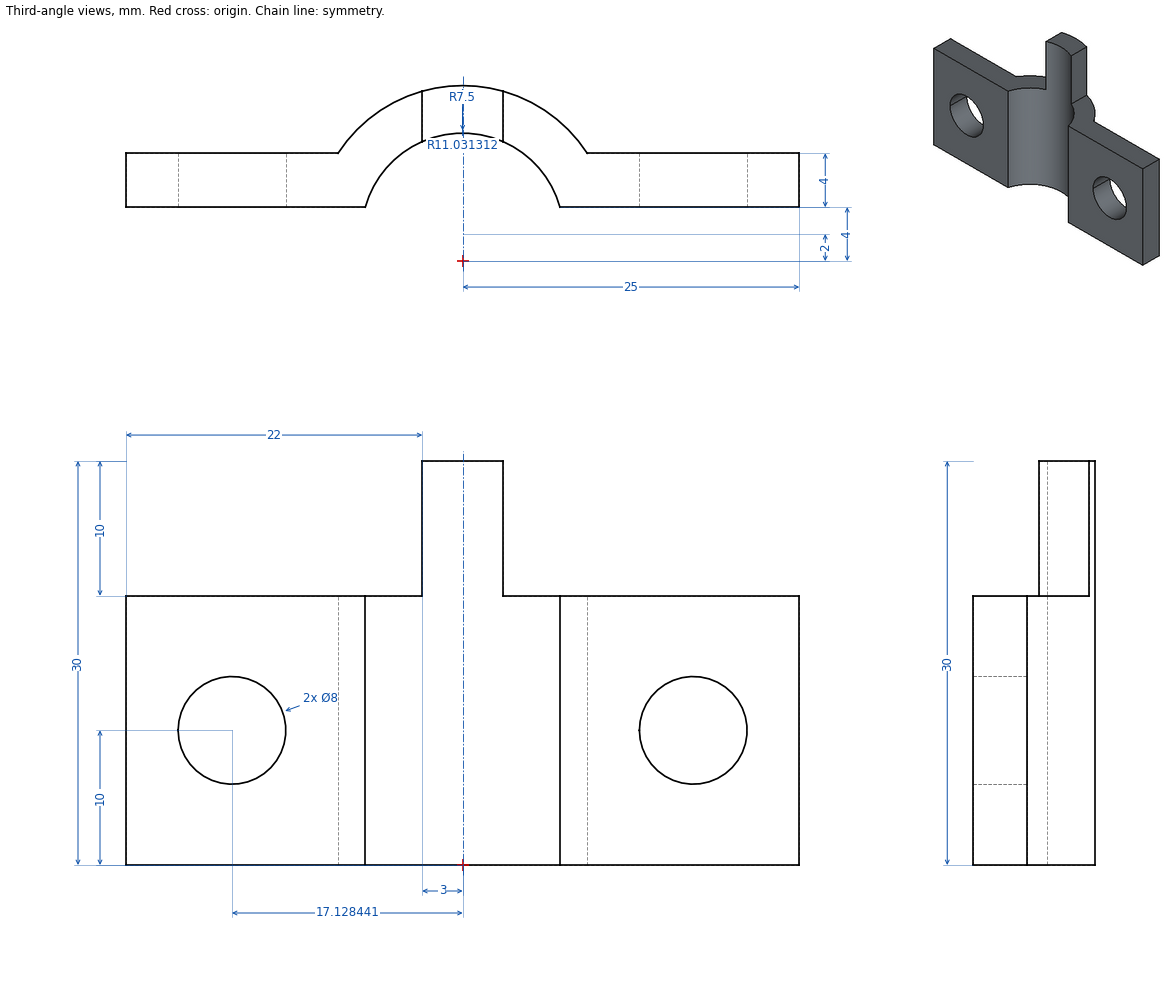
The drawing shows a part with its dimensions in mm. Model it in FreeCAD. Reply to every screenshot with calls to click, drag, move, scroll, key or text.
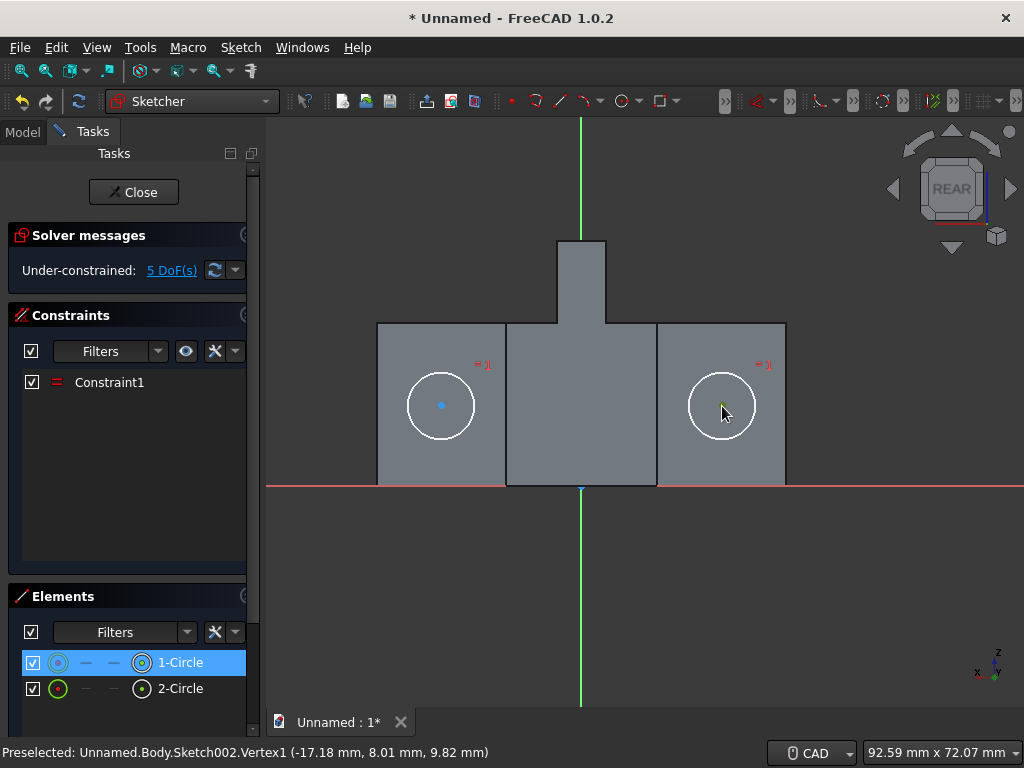
click(441, 406)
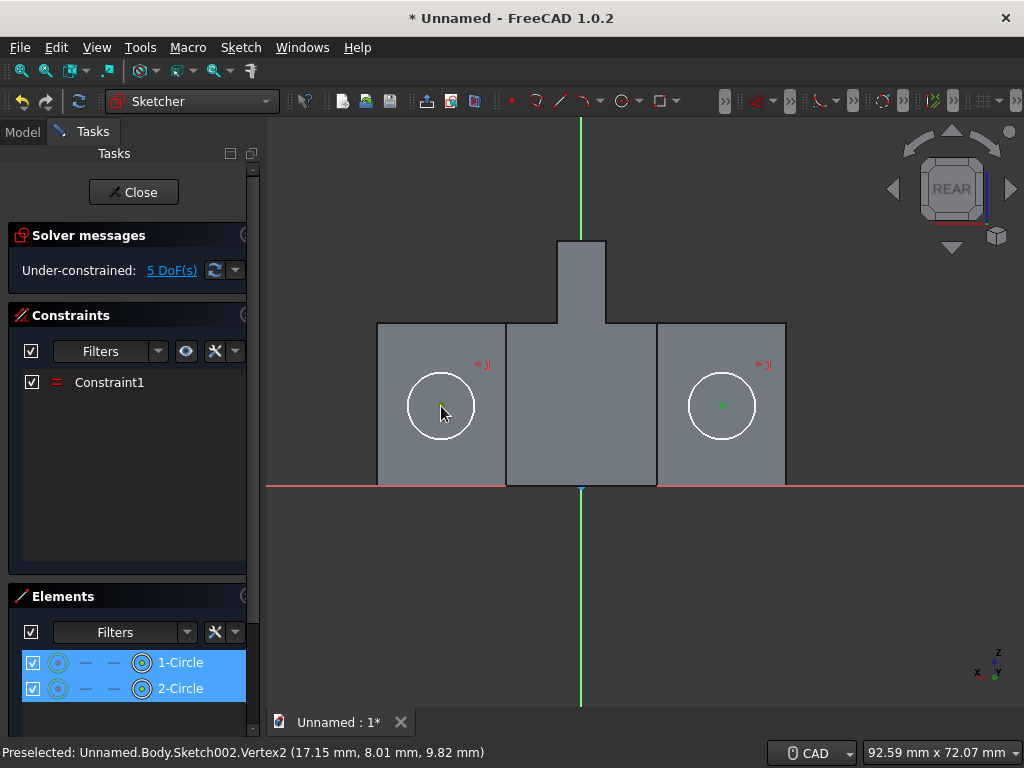
click(581, 641)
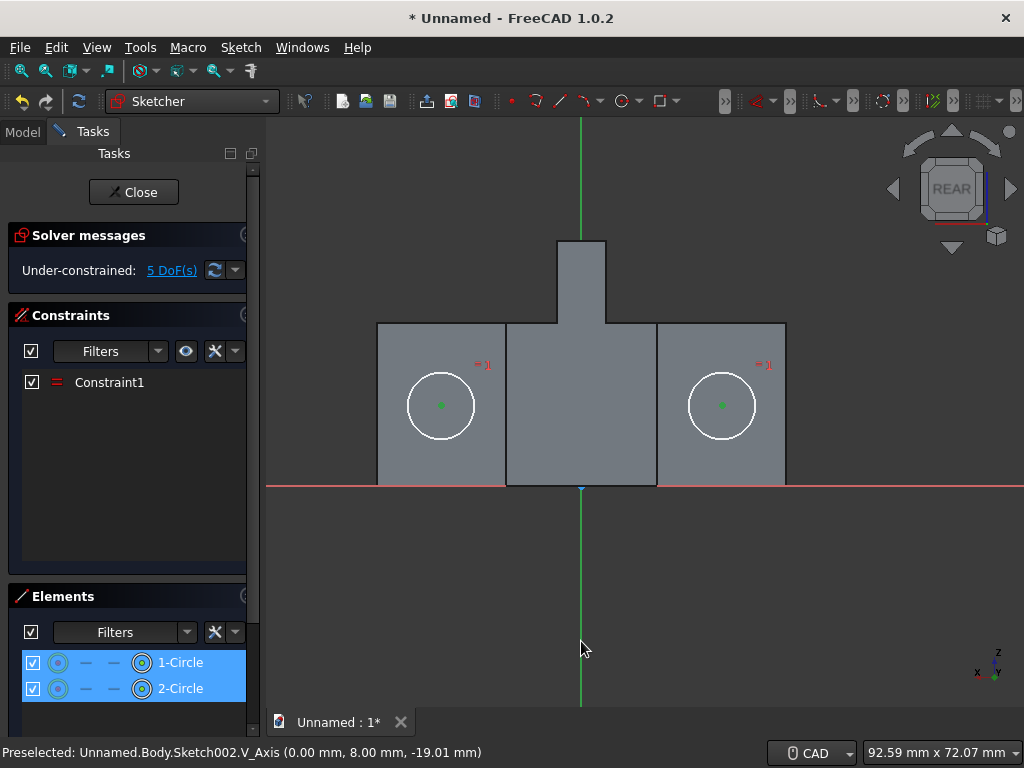
key(s)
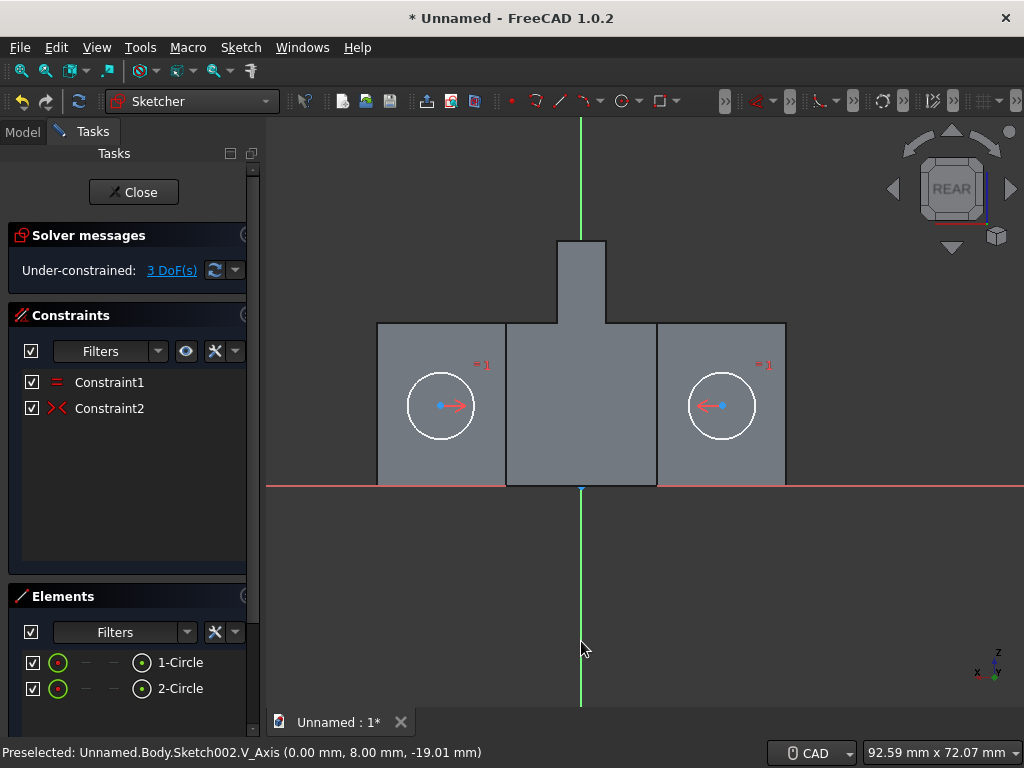
click(756, 102)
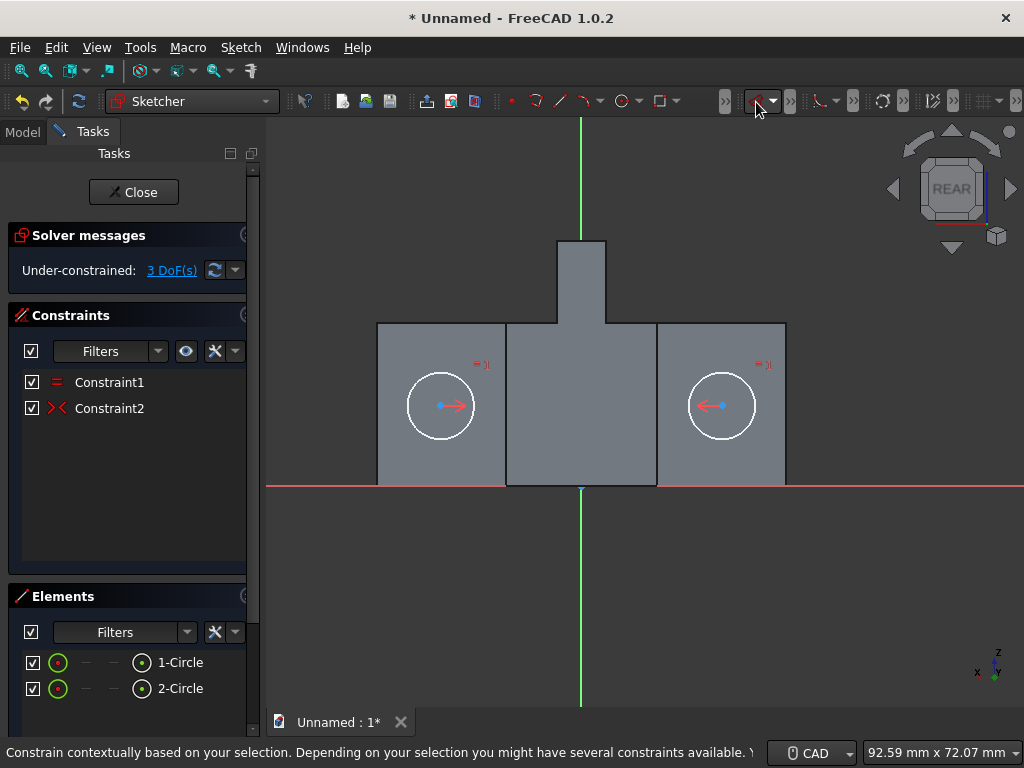
click(745, 382)
click(767, 359)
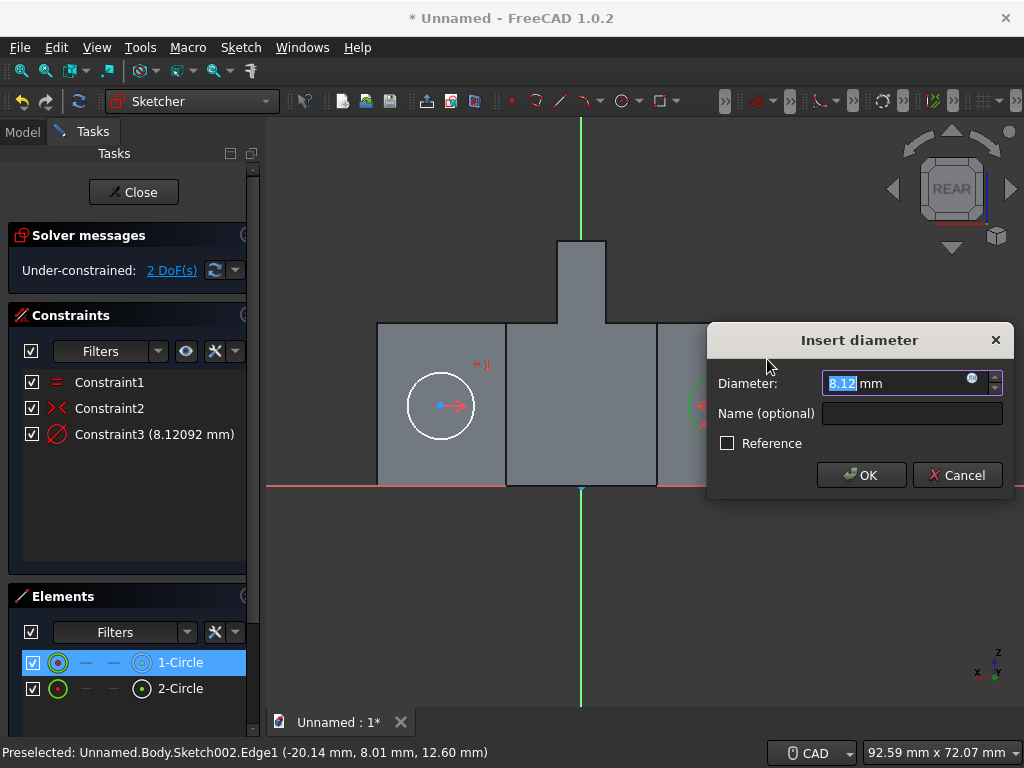
text(8)
key(Return)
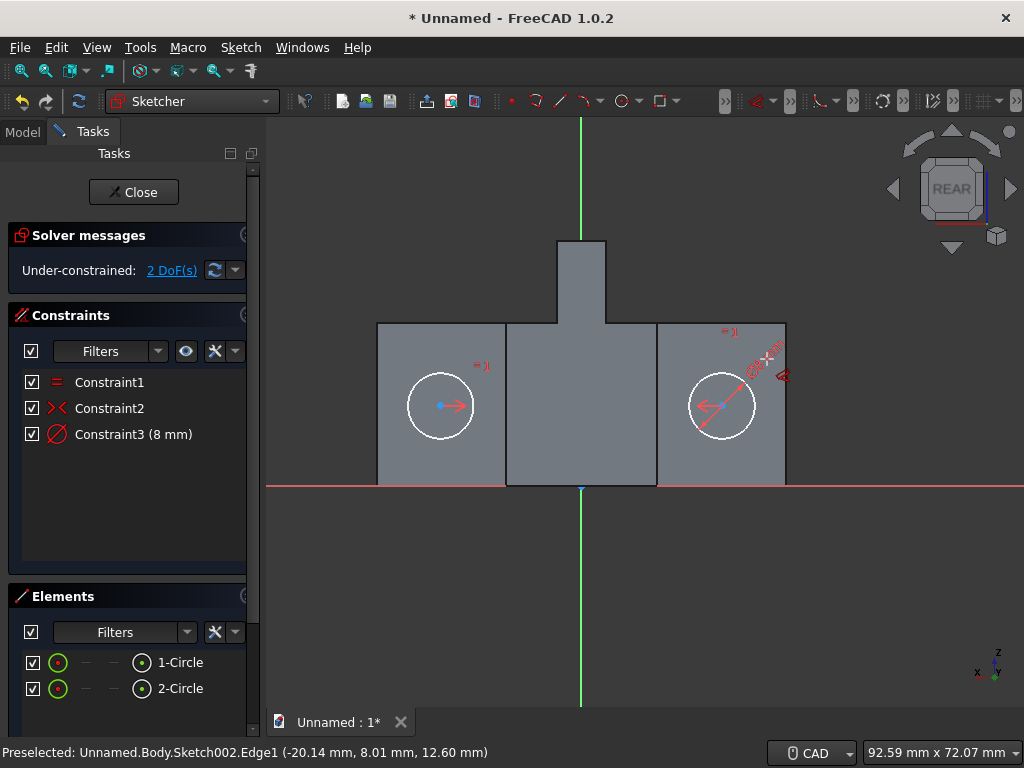
click(722, 406)
click(756, 446)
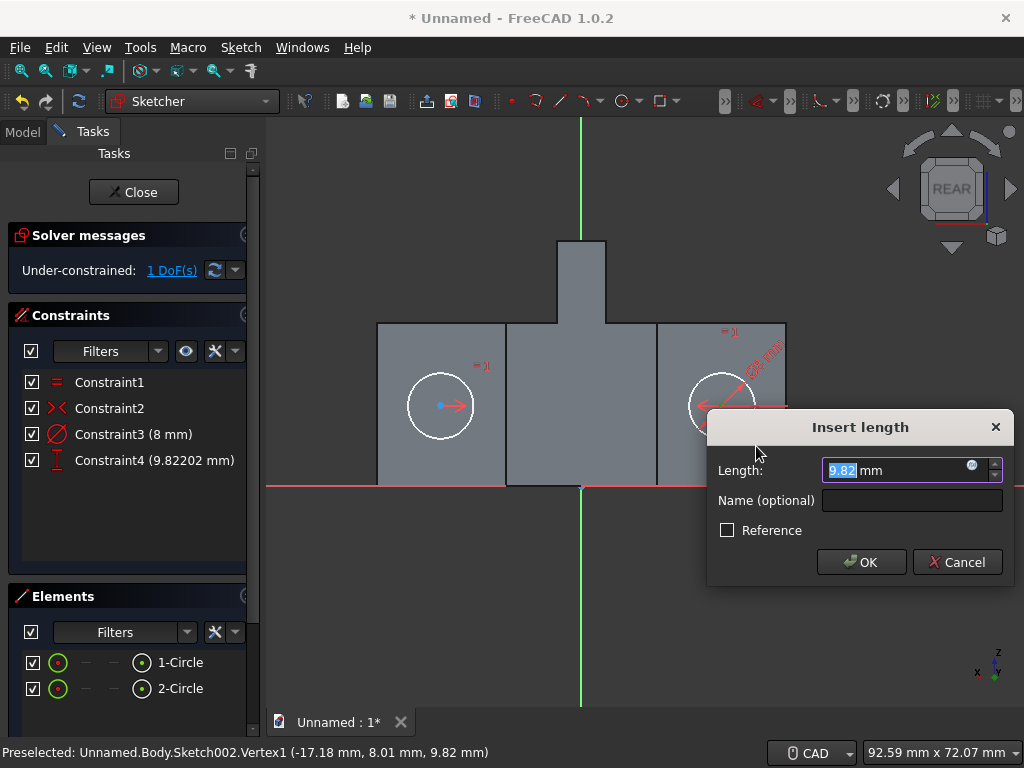
text(10)
key(Return)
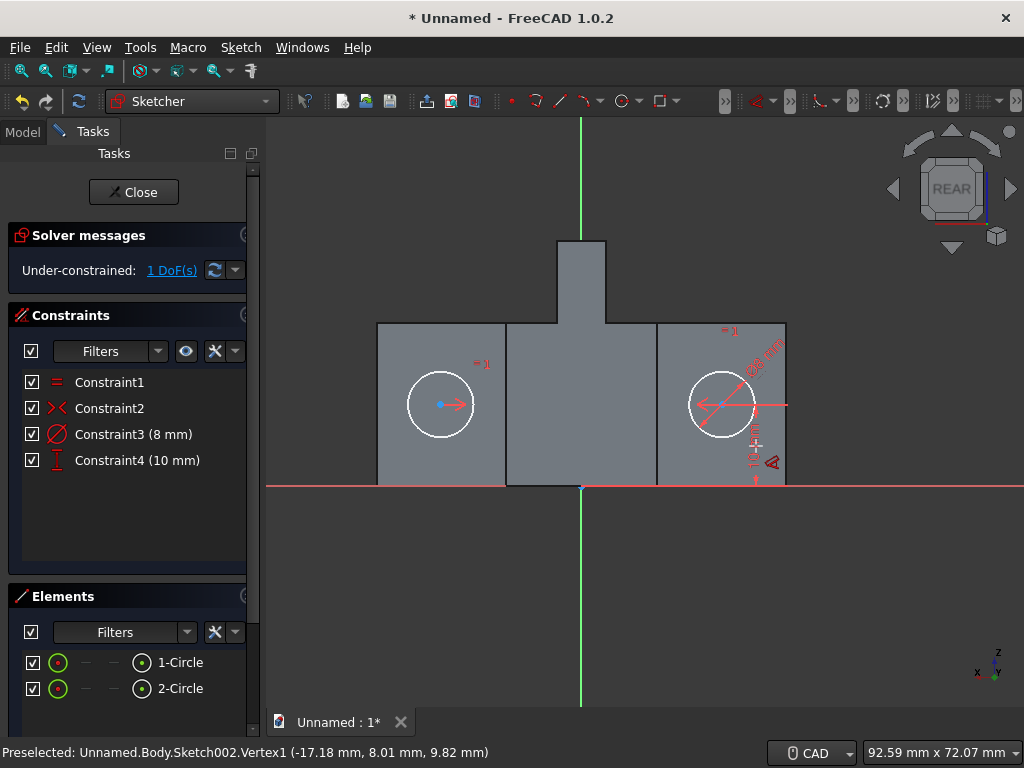
click(722, 405)
click(652, 520)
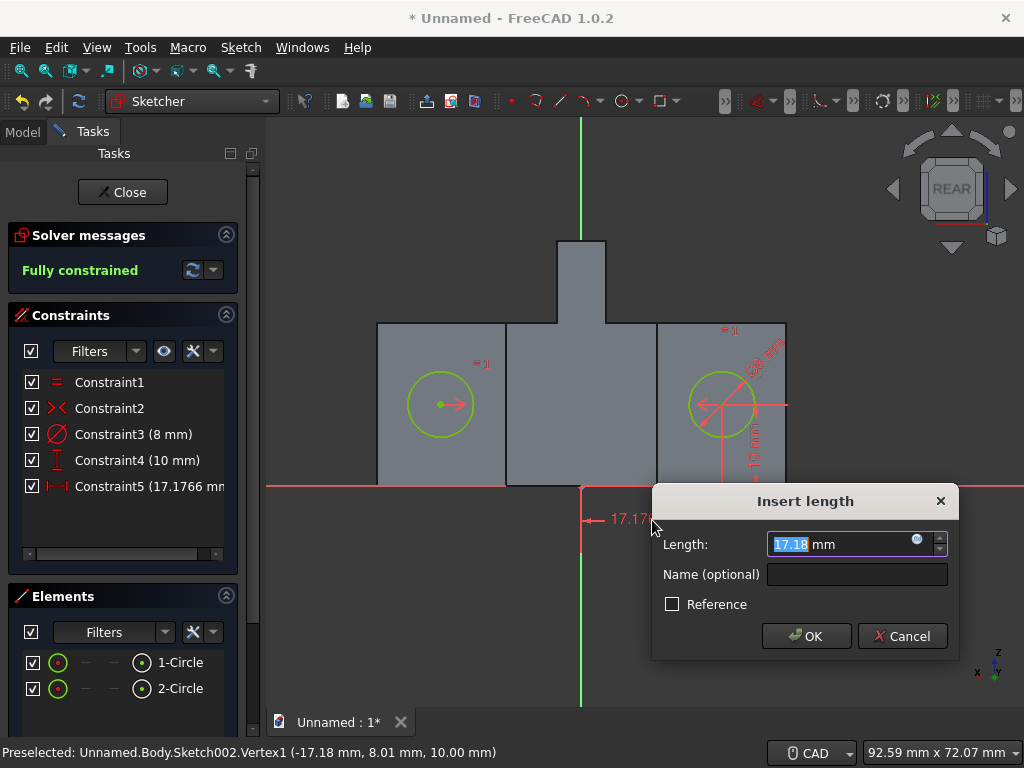
text(17.128441)
key(Return)
key(Escape)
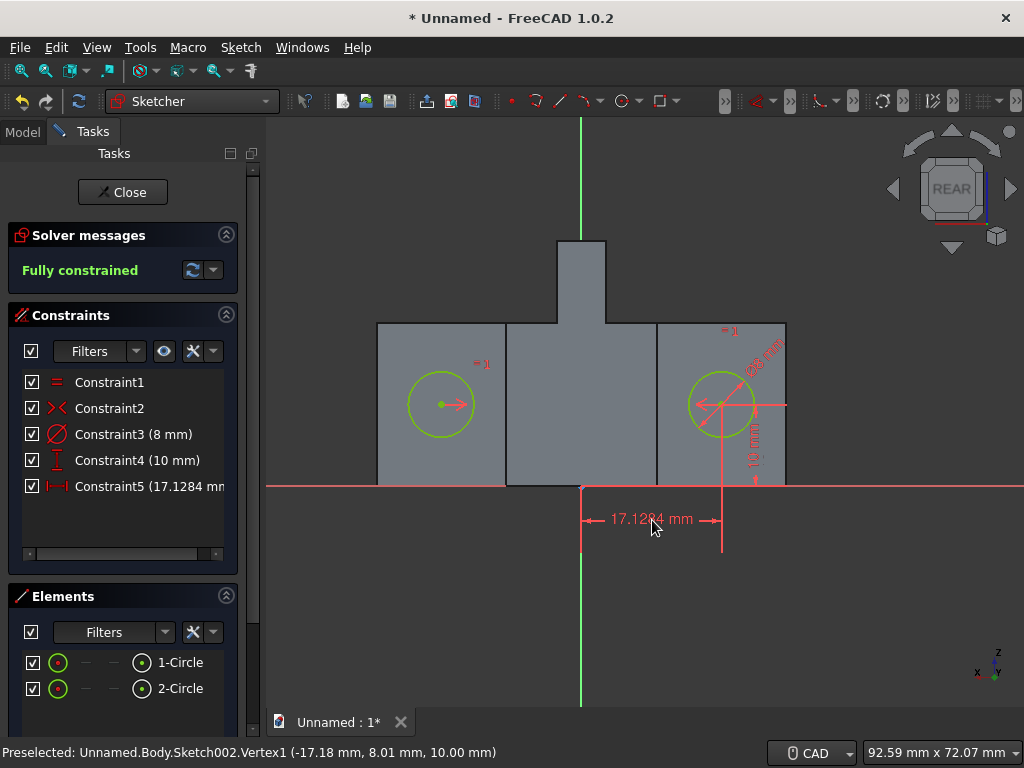
click(123, 192)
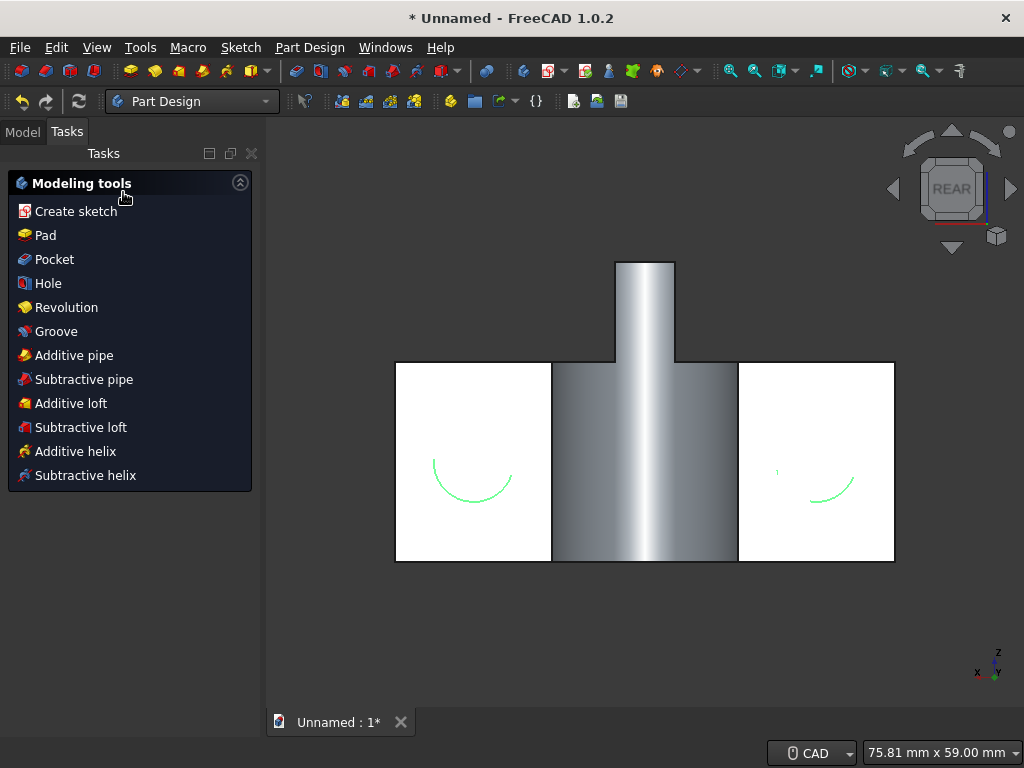
click(298, 72)